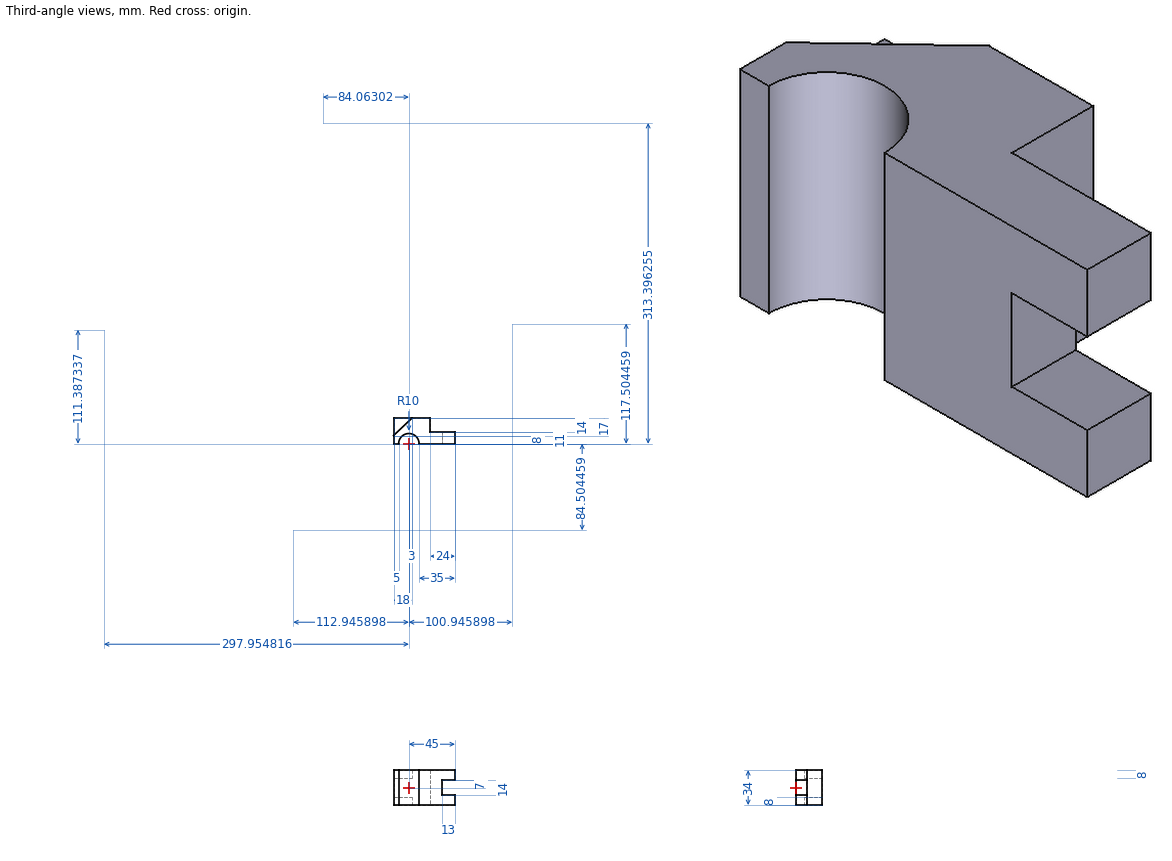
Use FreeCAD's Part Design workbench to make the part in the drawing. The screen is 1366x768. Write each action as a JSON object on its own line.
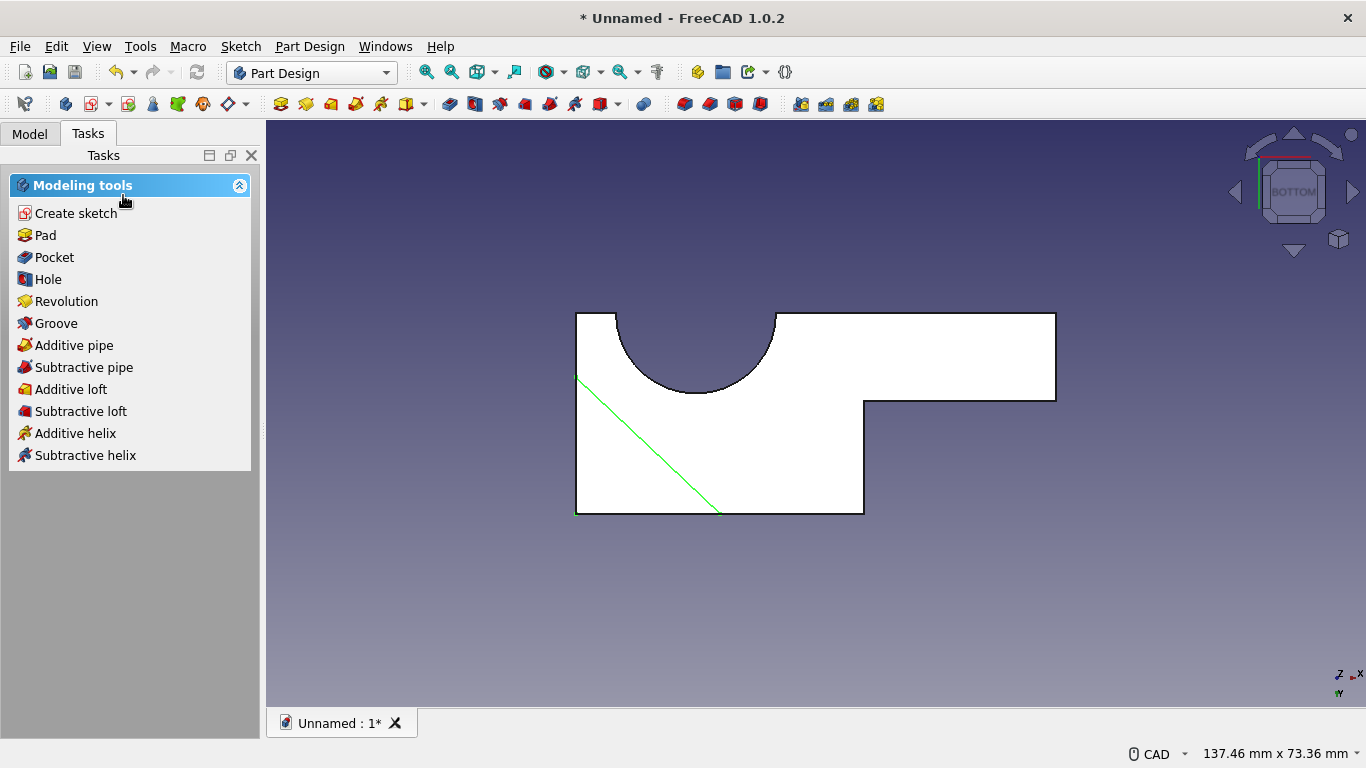
{"action": "left_click", "coordinate": [450, 104]}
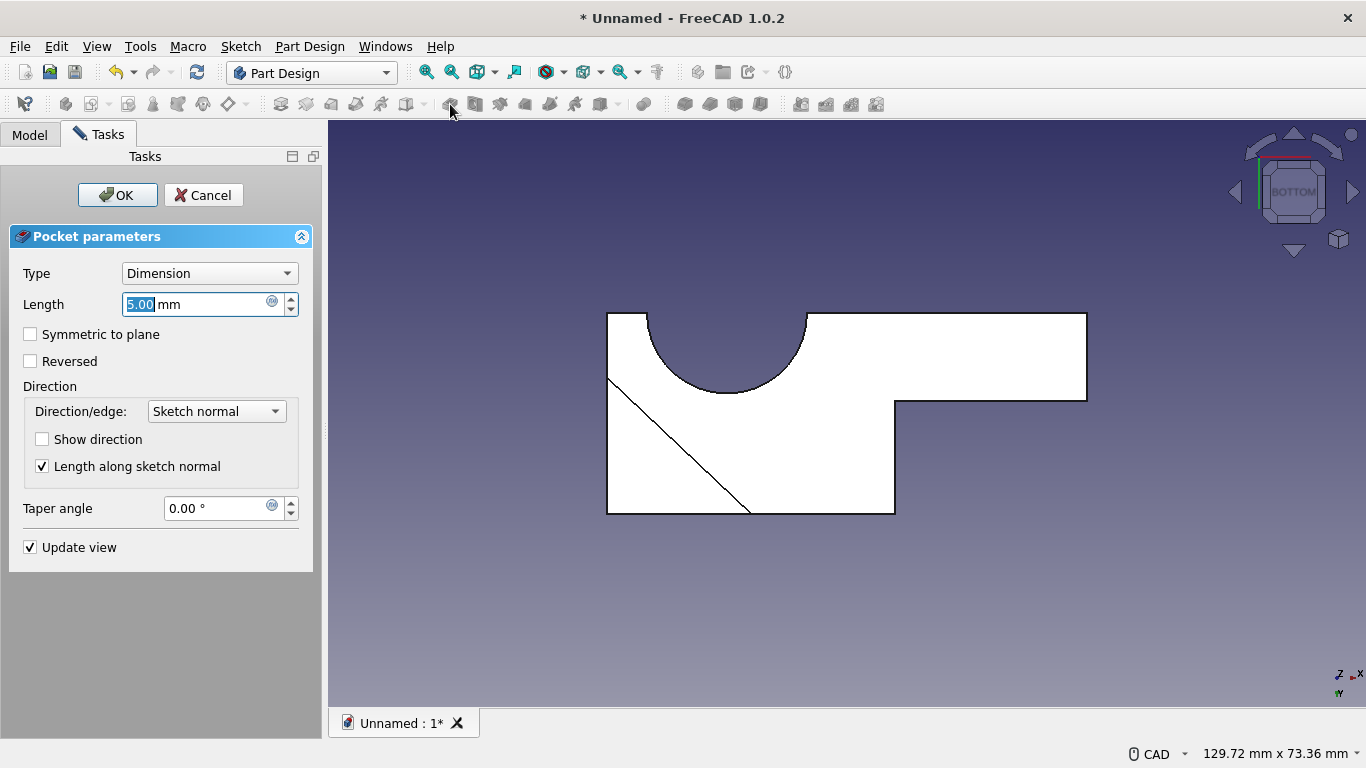
{"action": "type", "text": "8"}
{"action": "key", "text": "Tab"}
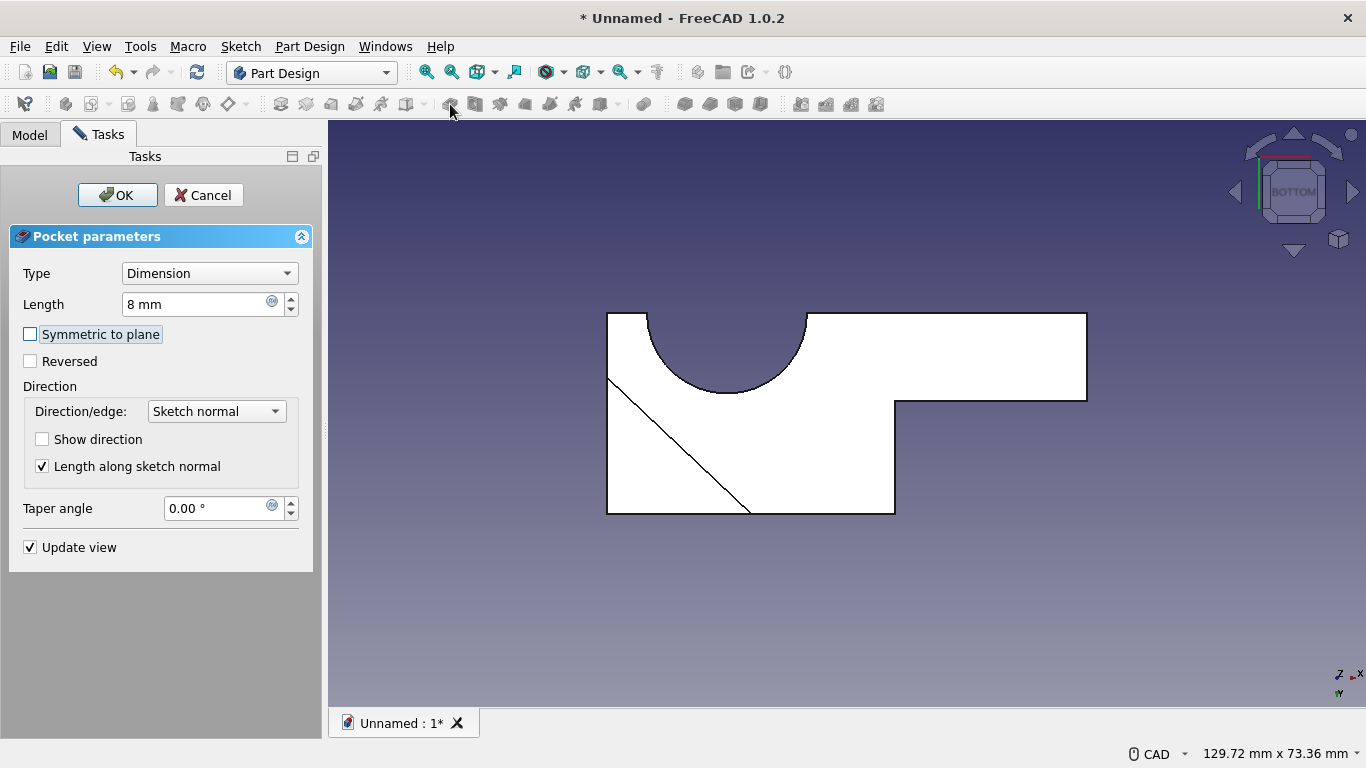
{"action": "left_click", "coordinate": [118, 195]}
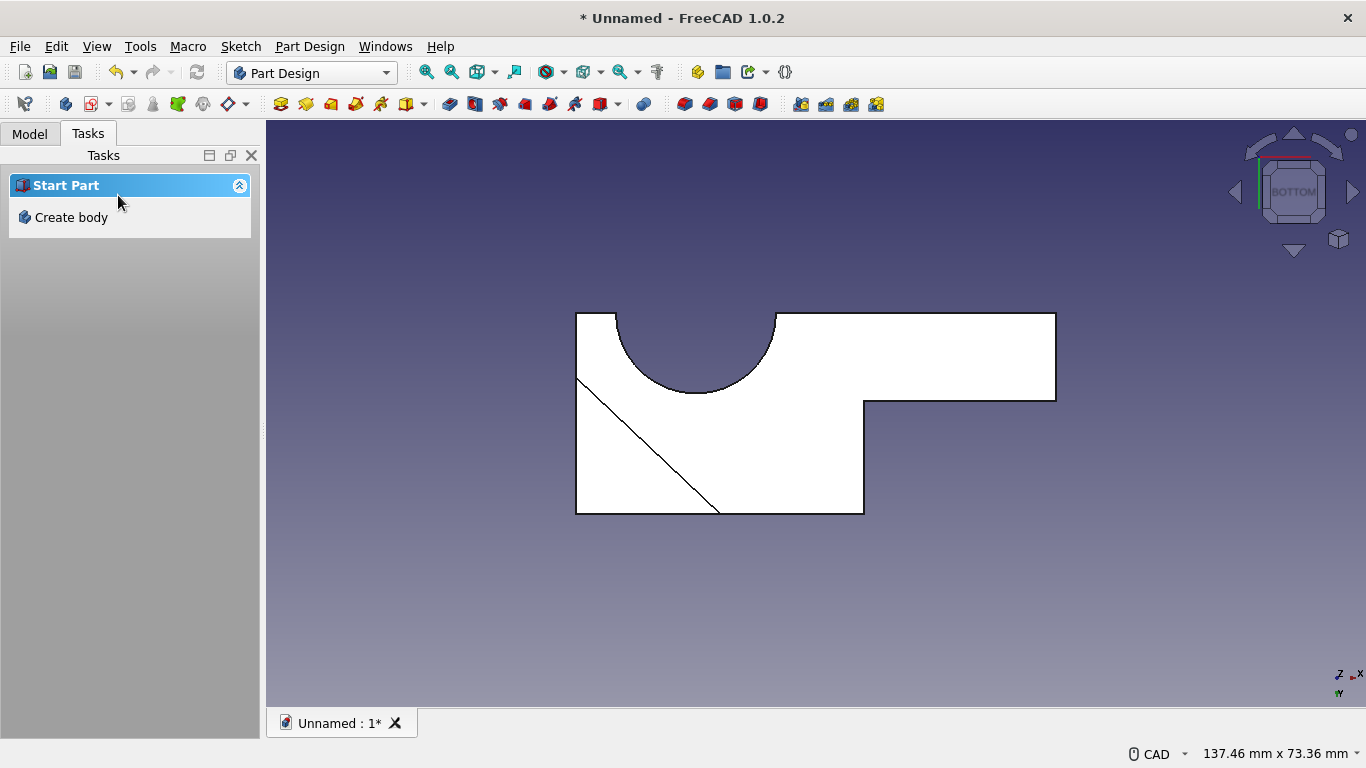
{"action": "key", "text": "0"}